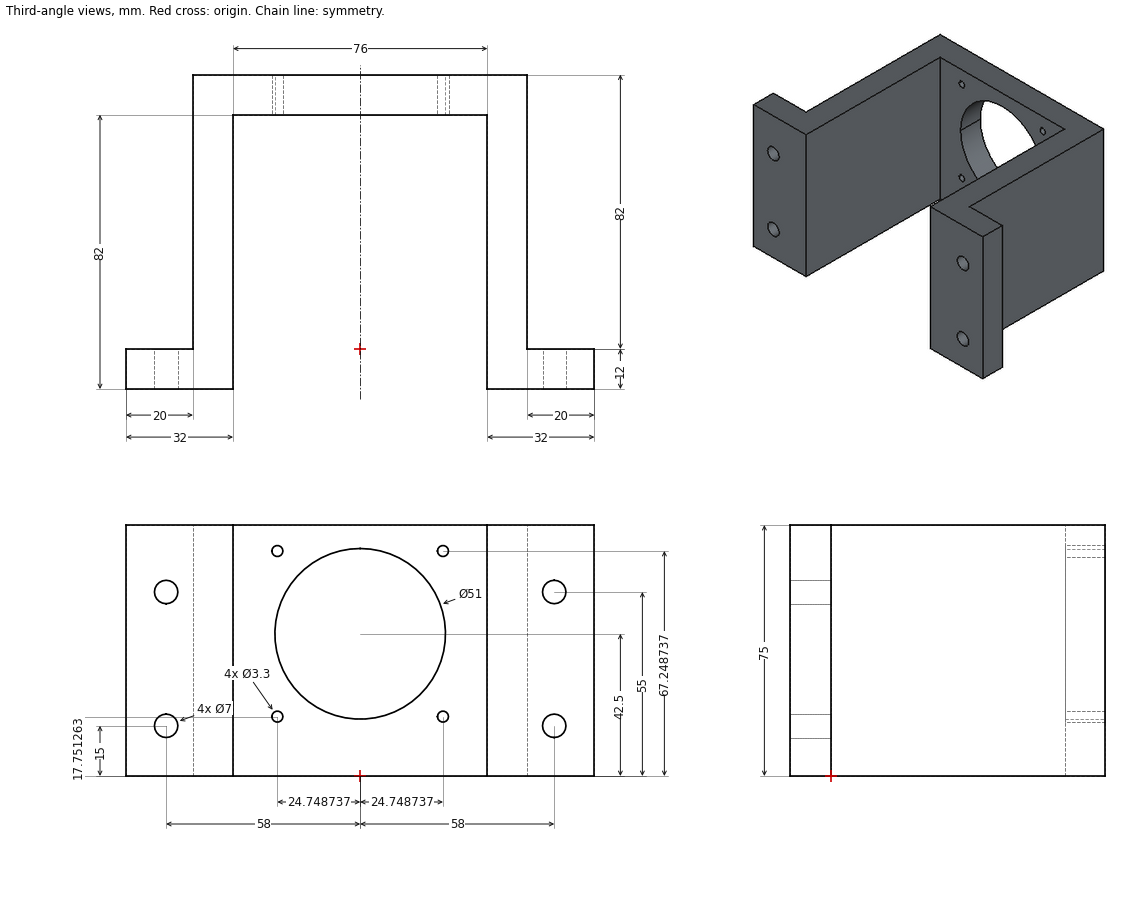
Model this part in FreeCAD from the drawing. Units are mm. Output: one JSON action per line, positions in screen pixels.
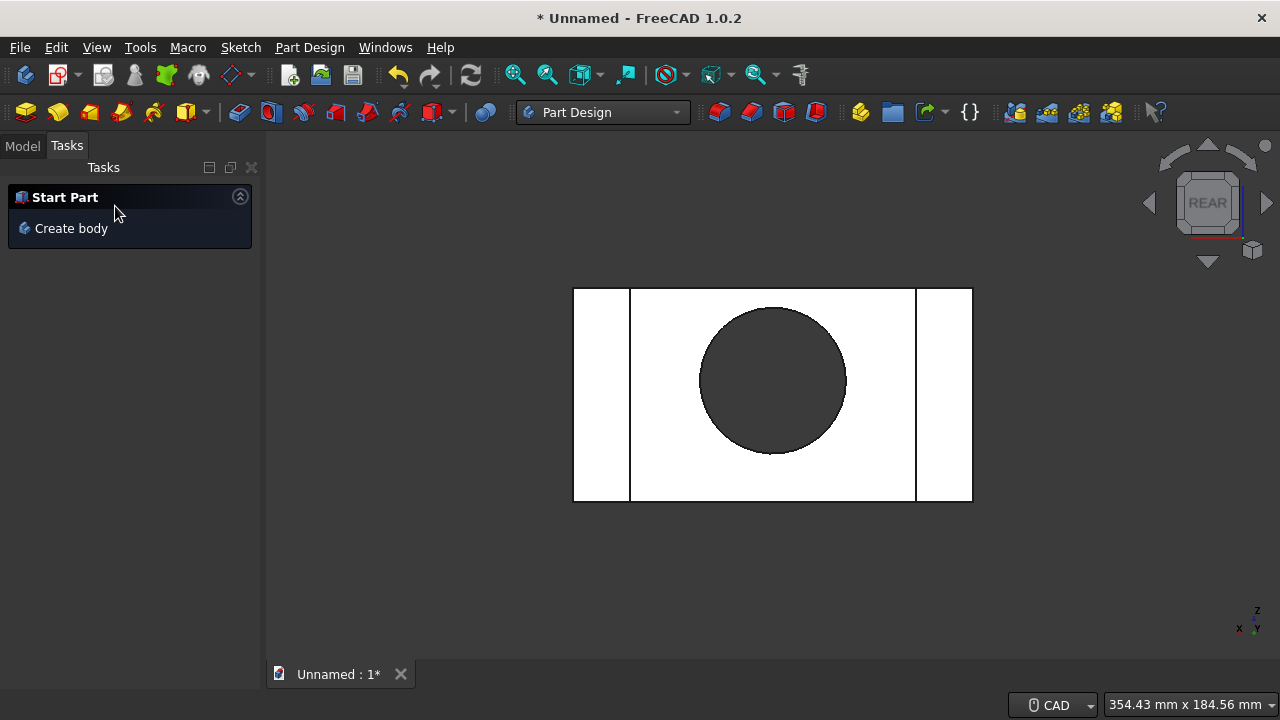
{"action": "left_click", "coordinate": [516, 76]}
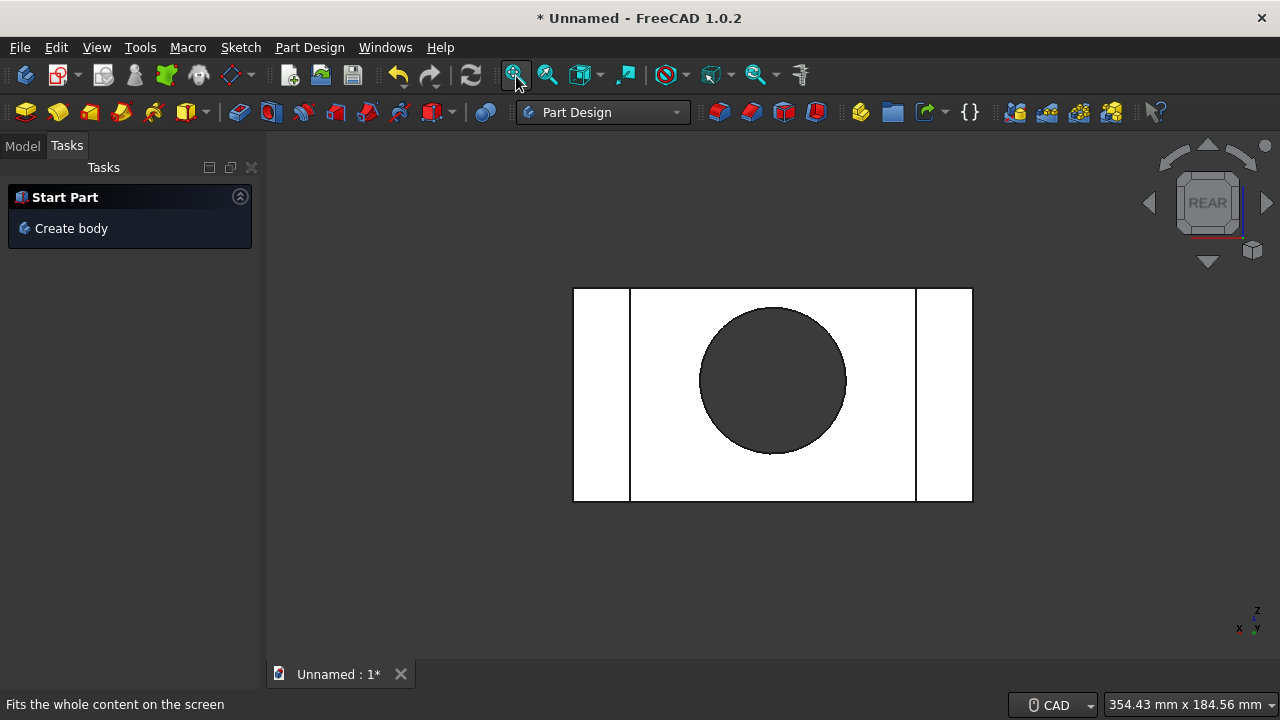
{"action": "left_click", "coordinate": [58, 76]}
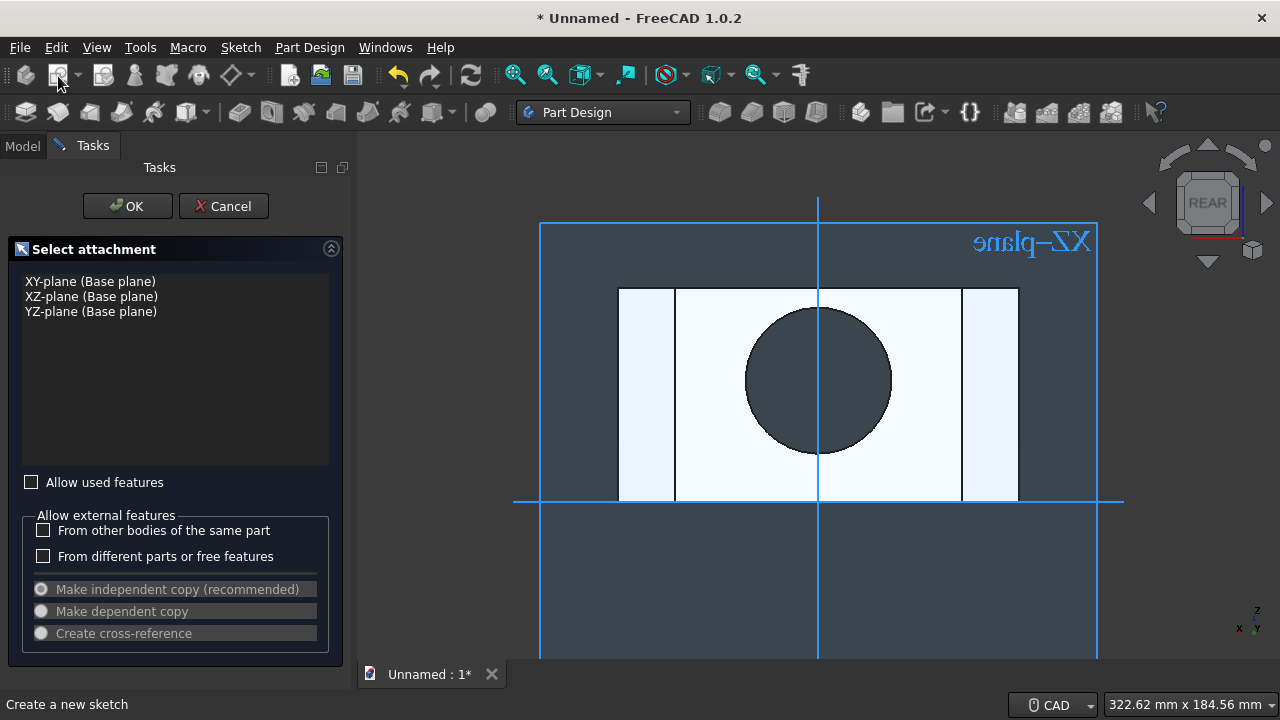
{"action": "left_click", "coordinate": [82, 296]}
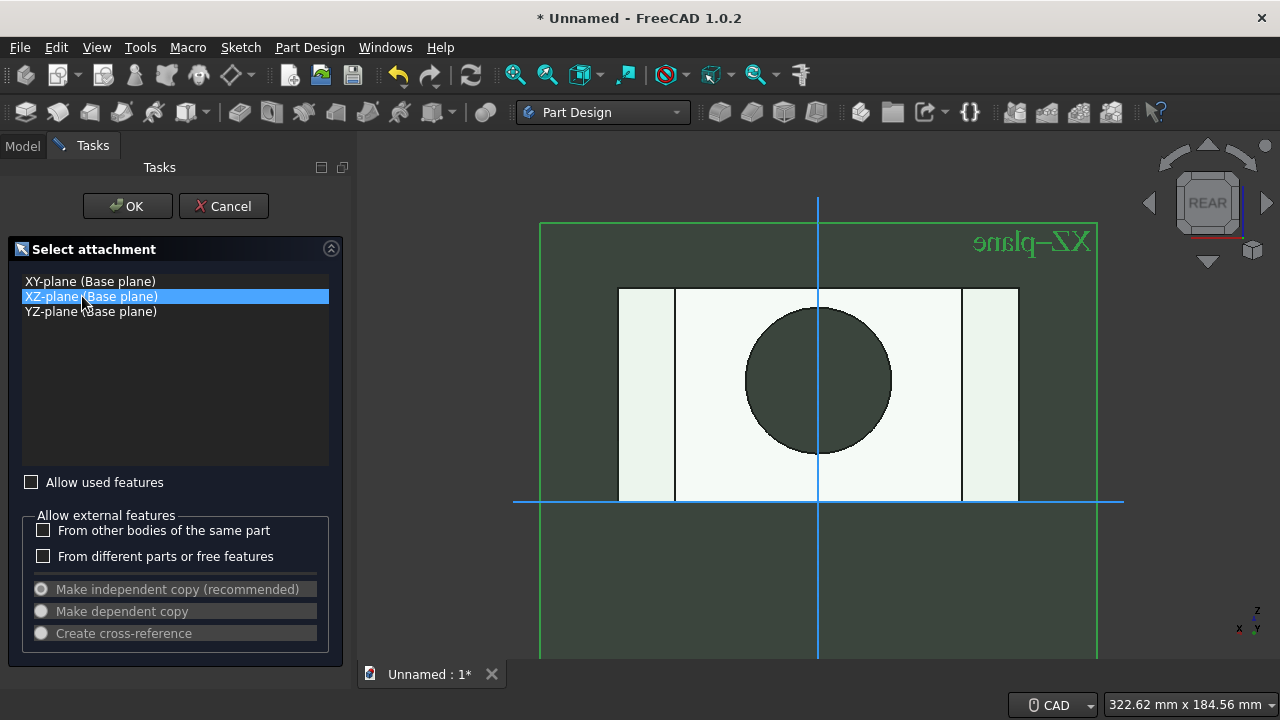
{"action": "left_click", "coordinate": [128, 206]}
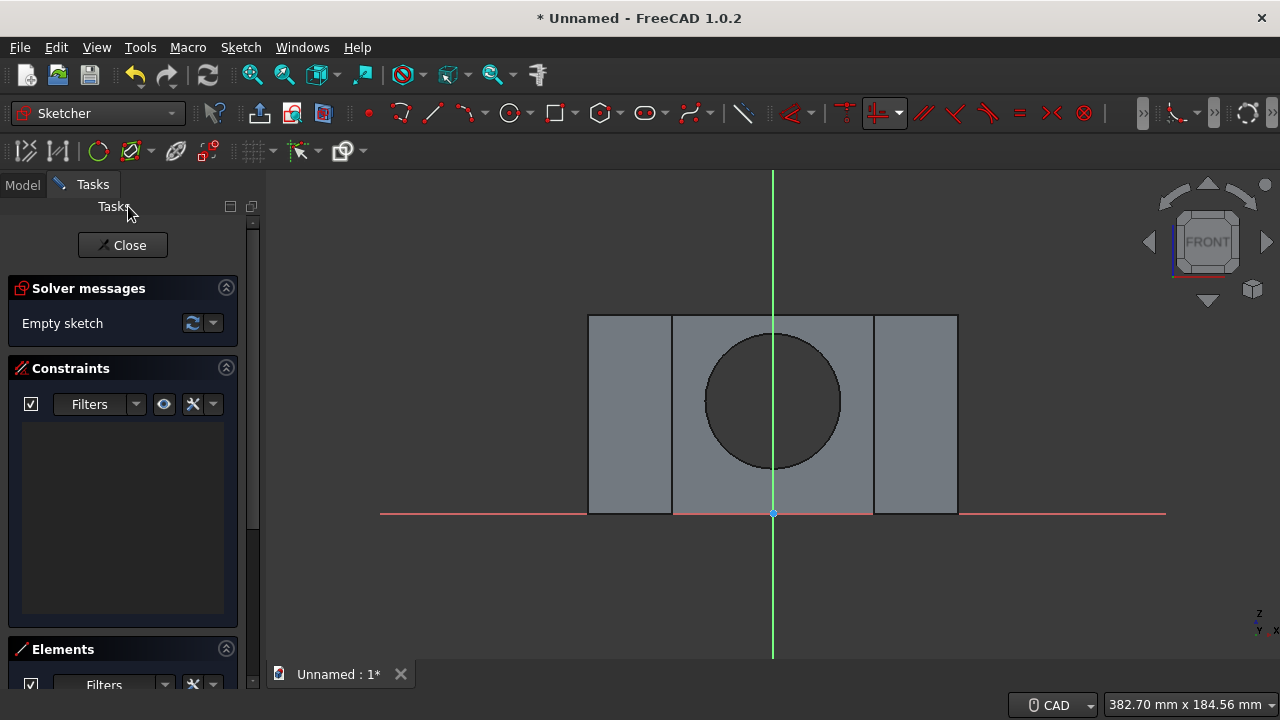
{"action": "left_click", "coordinate": [324, 114]}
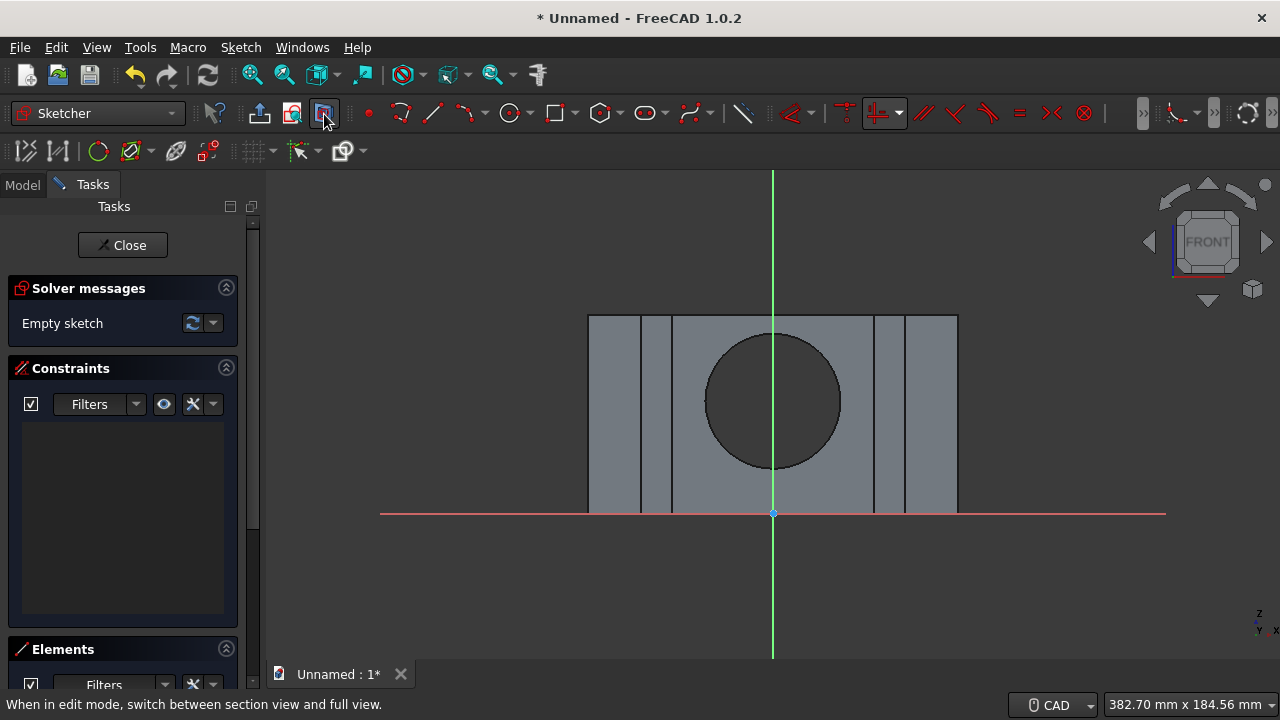
{"action": "scroll", "coordinate": [856, 463], "scroll_direction": "up", "scroll_amount": 3}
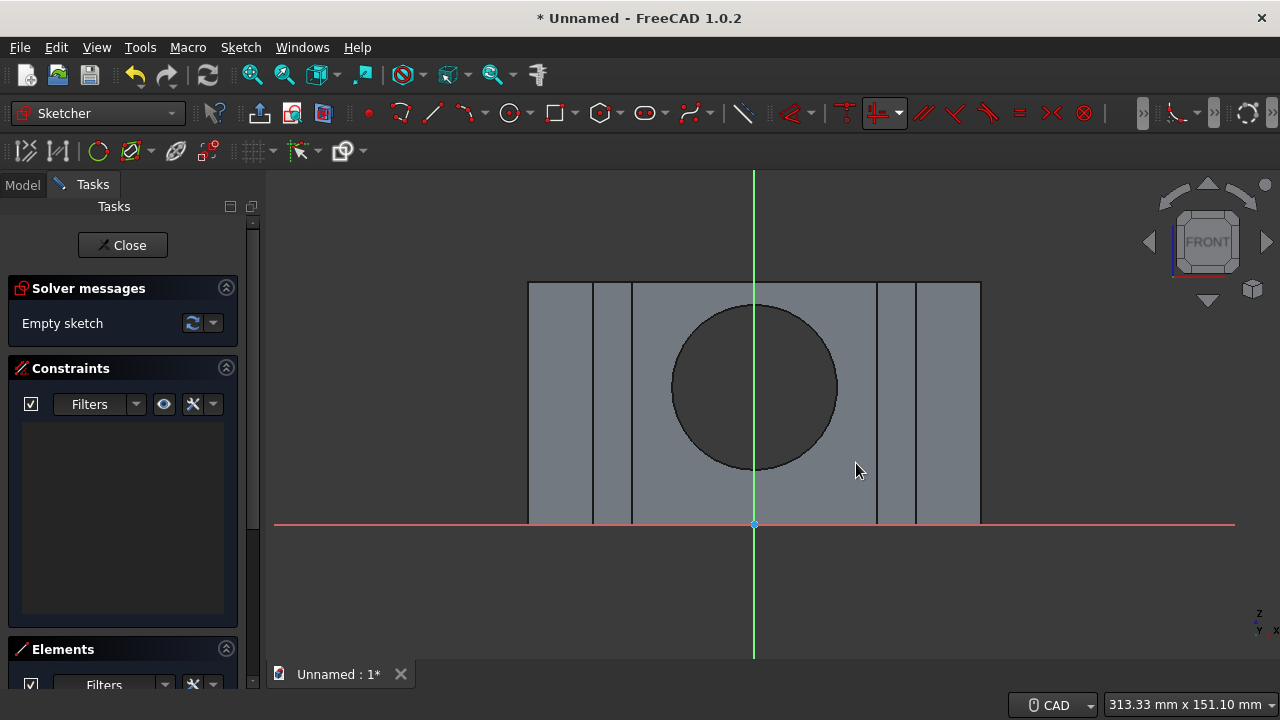
{"action": "left_click", "coordinate": [510, 114]}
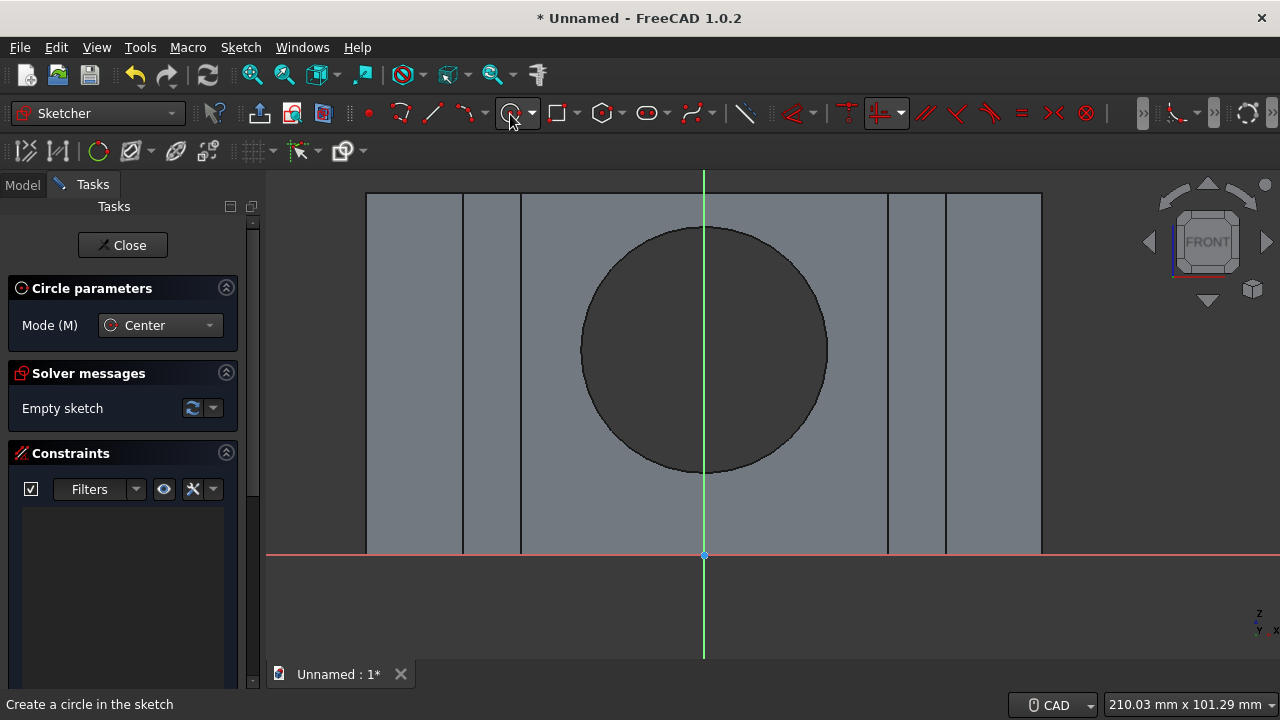
{"action": "scroll", "coordinate": [424, 483], "scroll_direction": "up", "scroll_amount": 2}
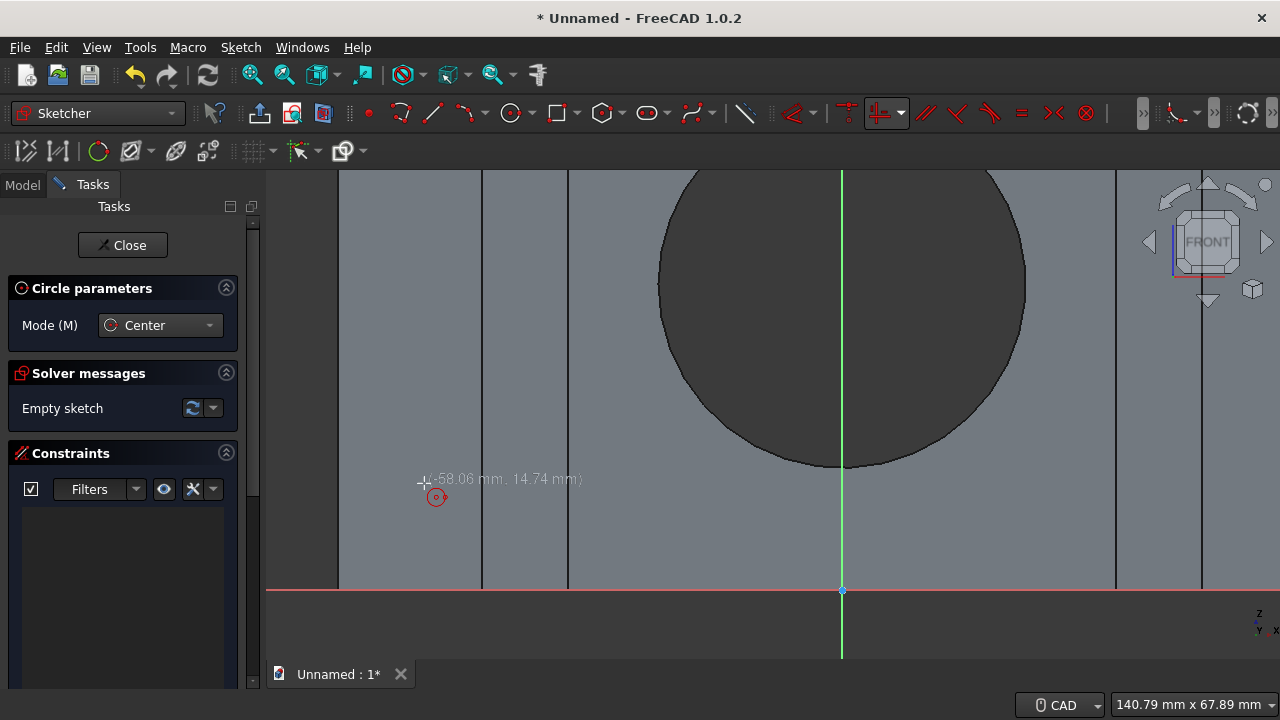
{"action": "left_click", "coordinate": [424, 482]}
{"action": "mouse_move", "coordinate": [442, 465]}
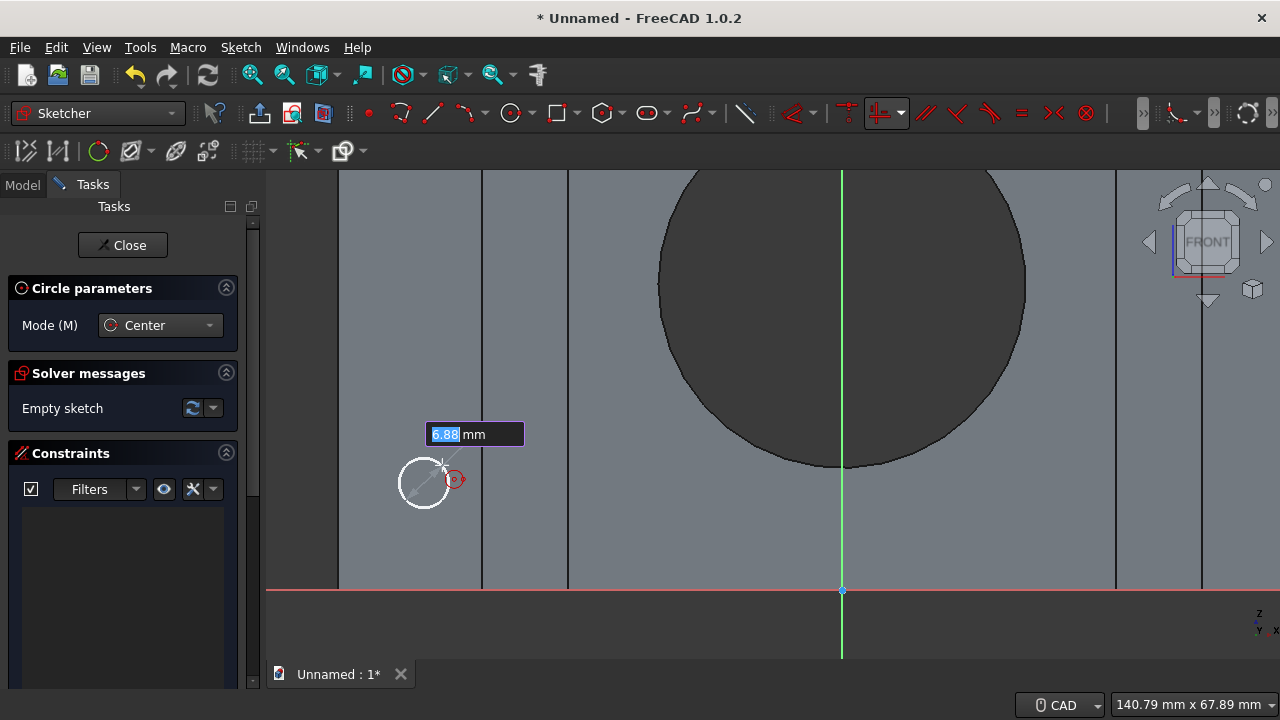
{"action": "type", "text": "7"}
{"action": "key", "text": "Return"}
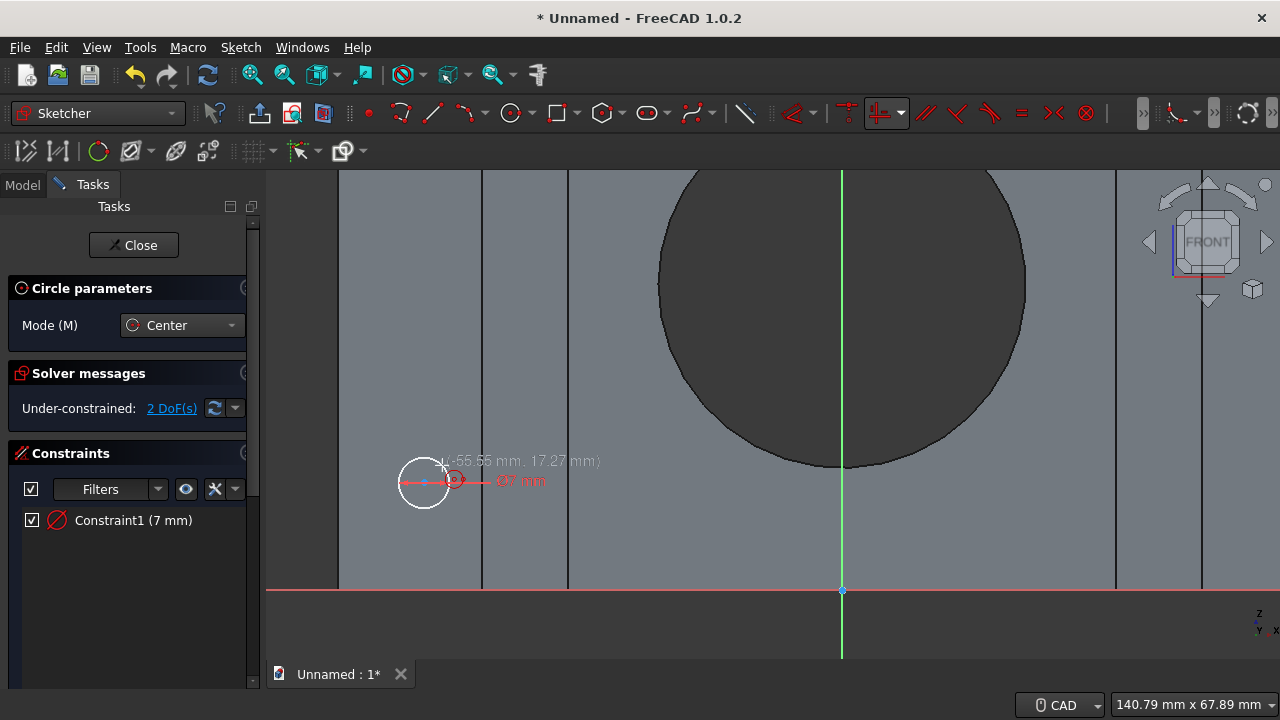
{"action": "scroll", "coordinate": [425, 485], "scroll_direction": "down", "scroll_amount": 2}